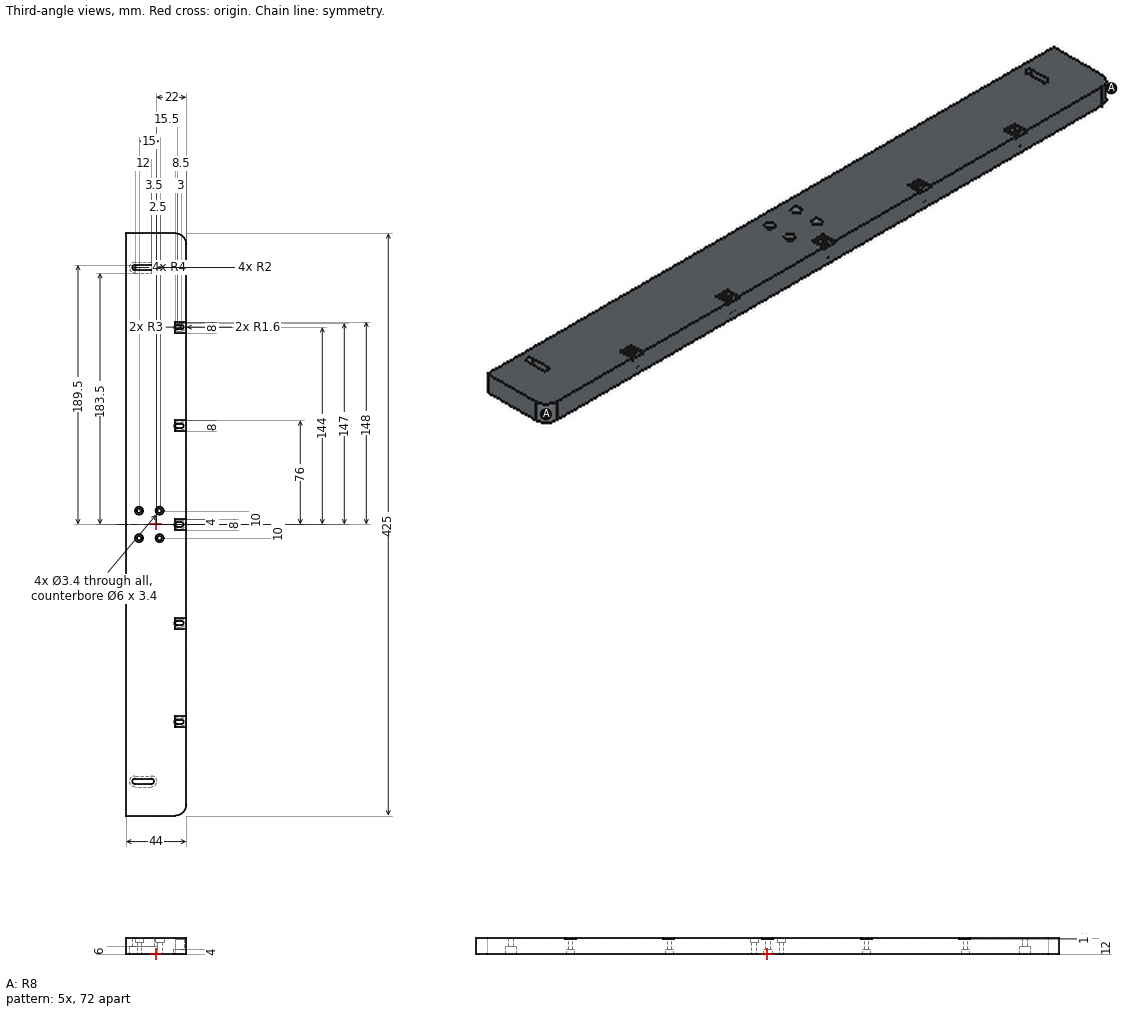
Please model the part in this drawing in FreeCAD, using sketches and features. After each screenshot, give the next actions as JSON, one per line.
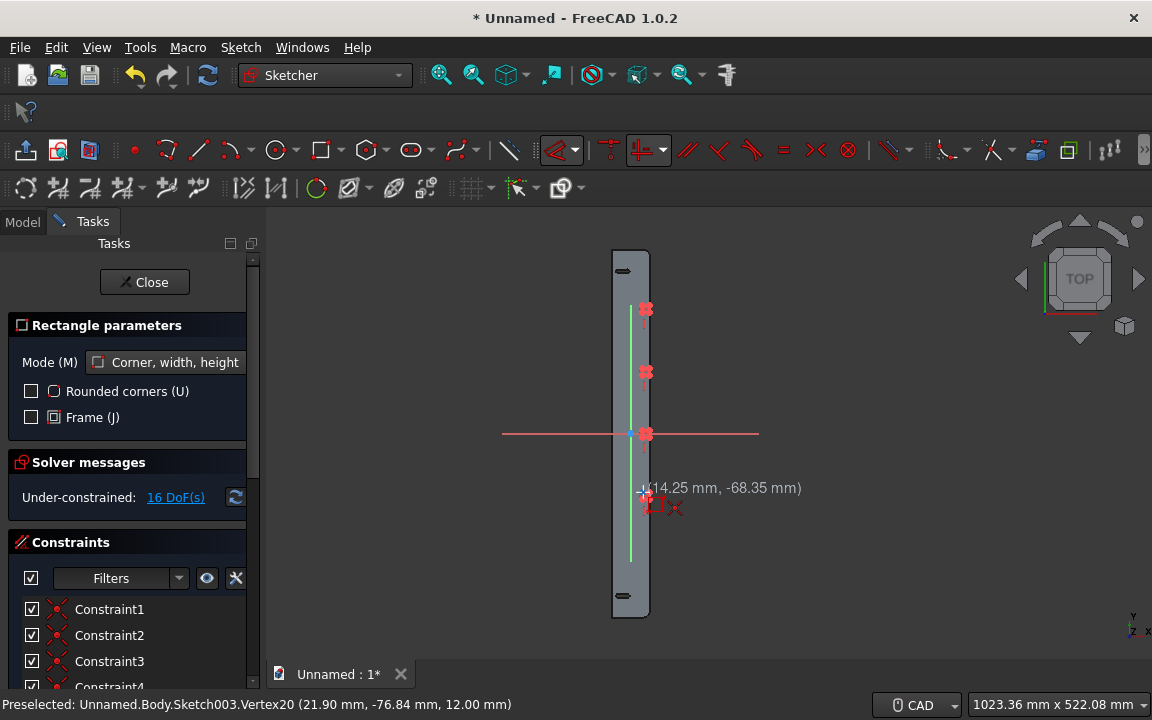
{"action": "scroll", "coordinate": [643, 555], "scroll_direction": "up", "scroll_amount": 5}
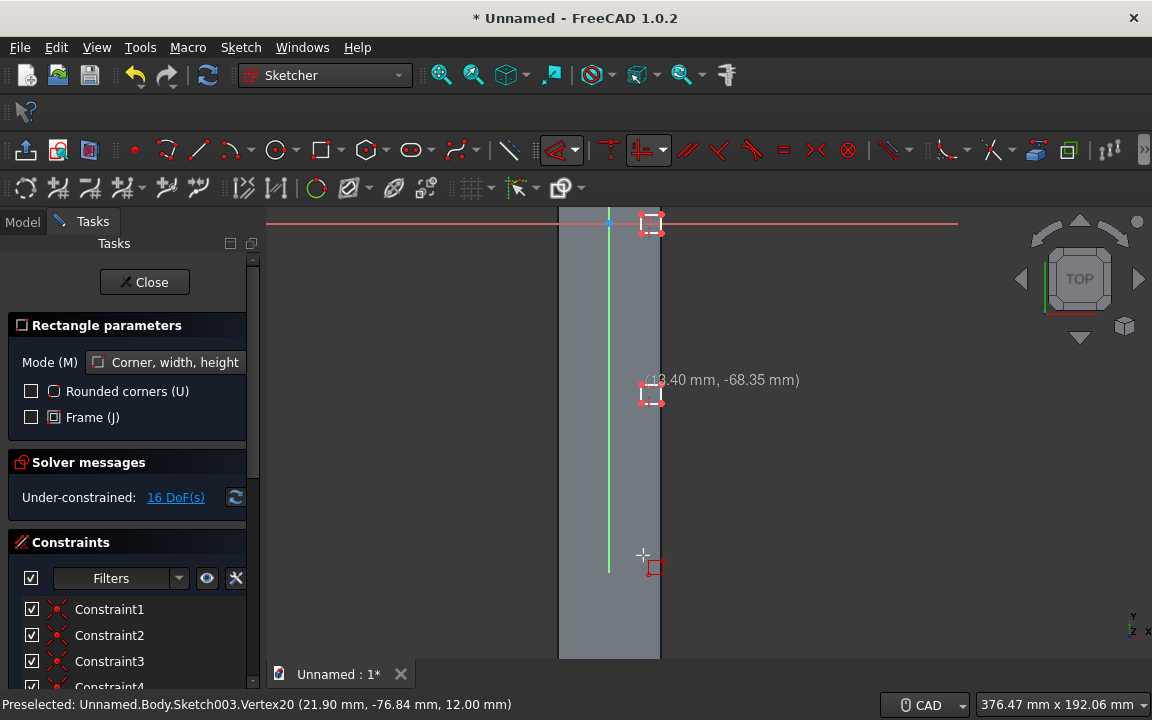
{"action": "left_click", "coordinate": [641, 553]}
{"action": "left_click", "coordinate": [661, 572]}
{"action": "key", "text": "Escape"}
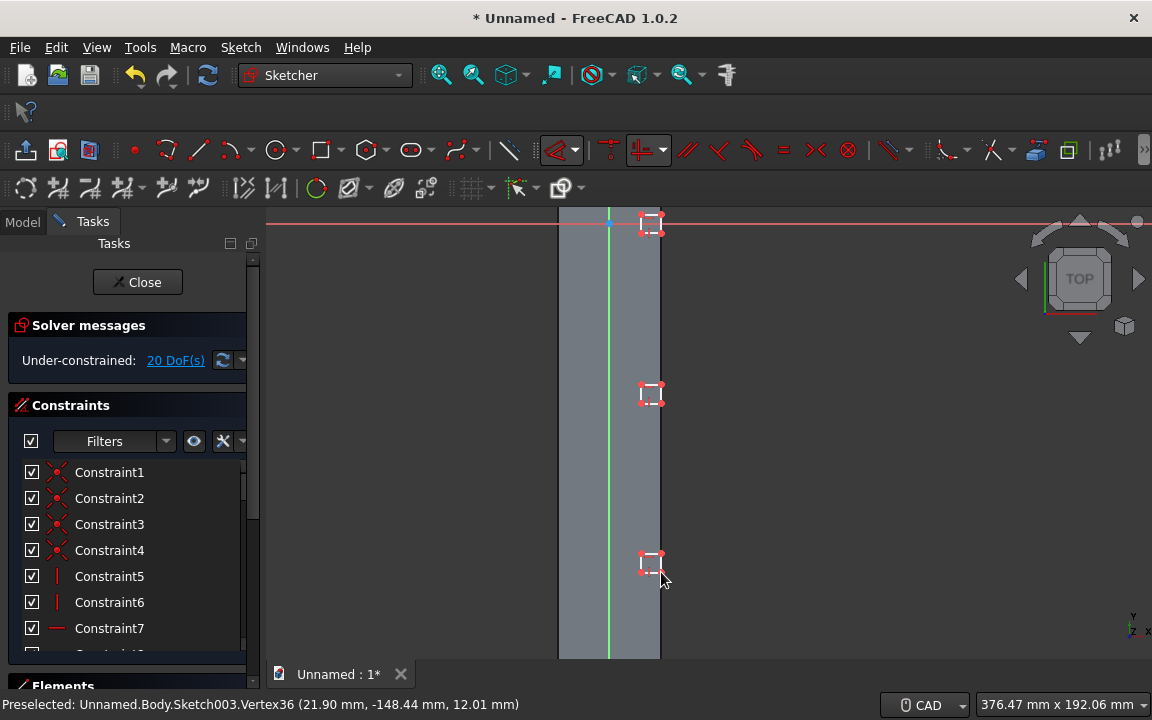
{"action": "scroll", "coordinate": [643, 555], "scroll_direction": "down", "scroll_amount": 5}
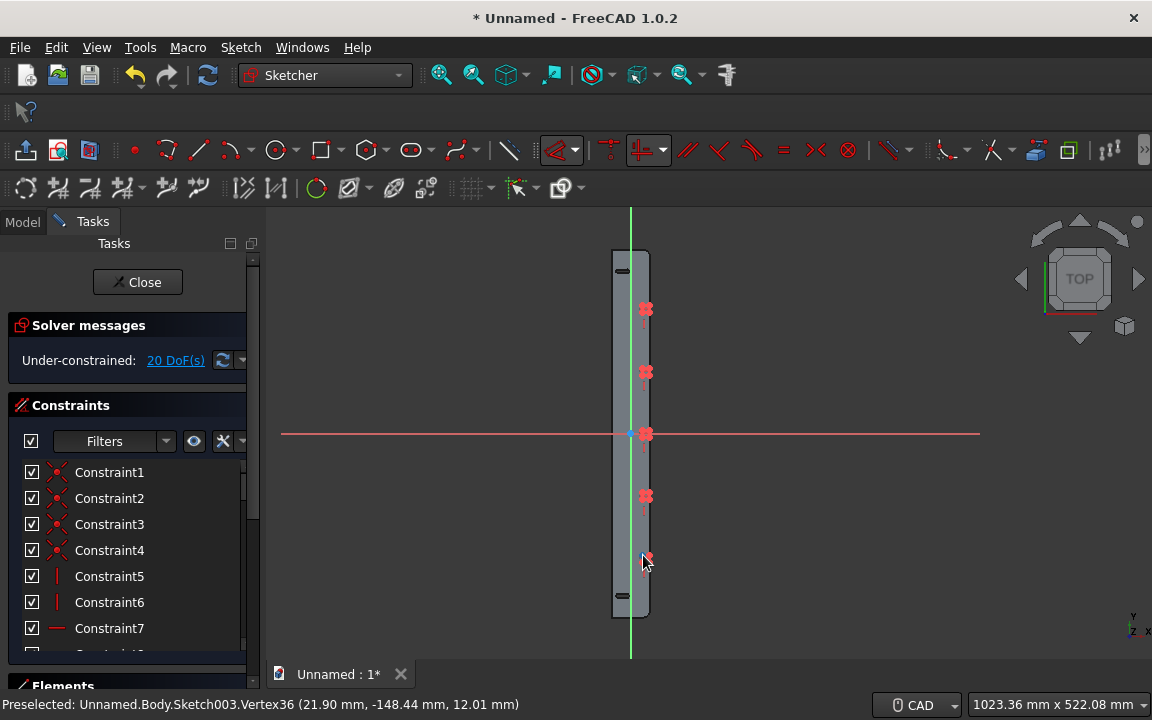
{"action": "scroll", "coordinate": [643, 375], "scroll_direction": "up", "scroll_amount": 3}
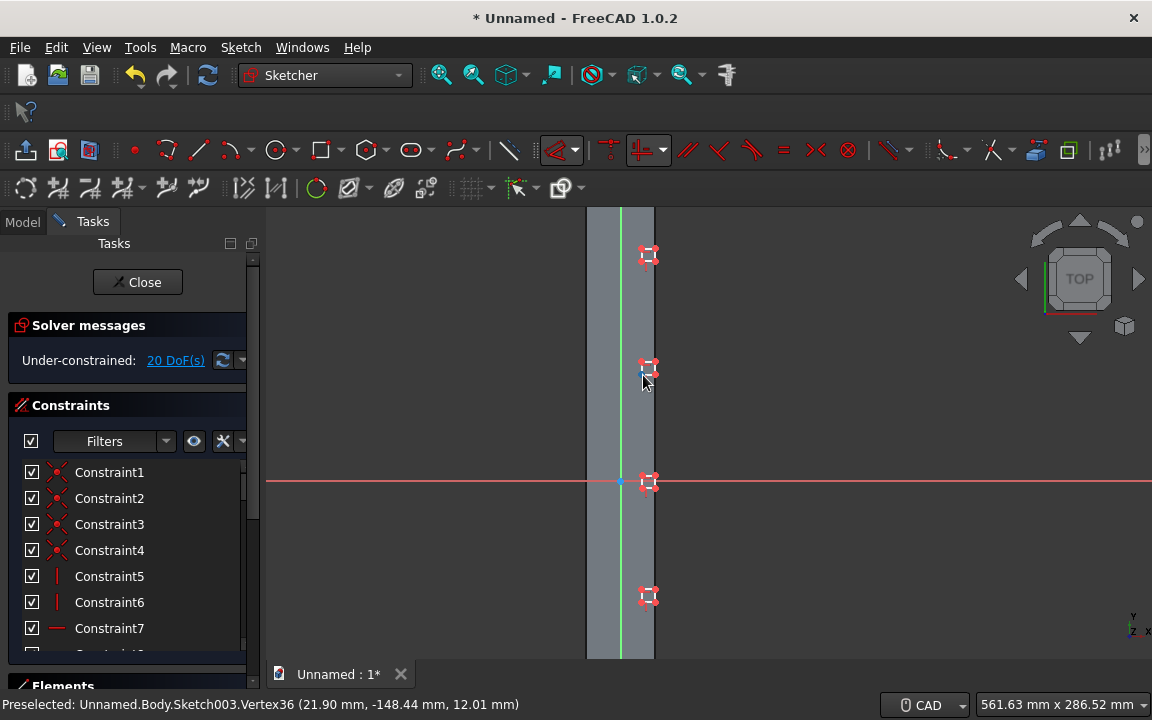
{"action": "left_click", "coordinate": [642, 375]}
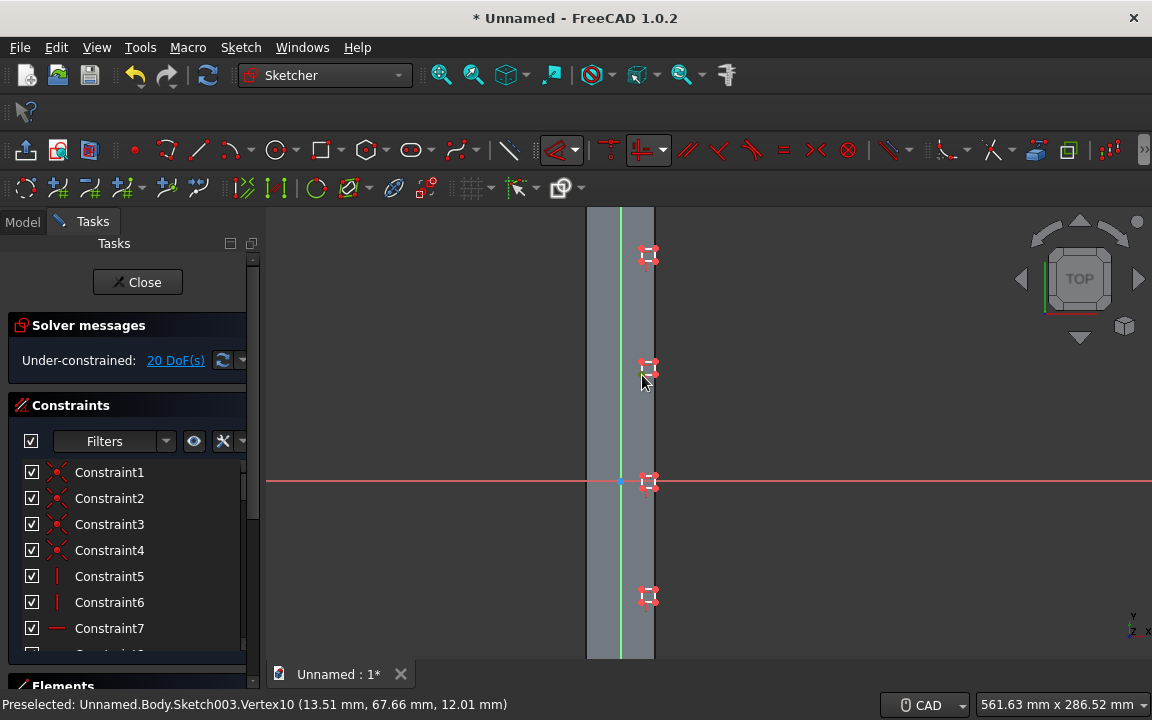
{"action": "left_click", "coordinate": [642, 589]}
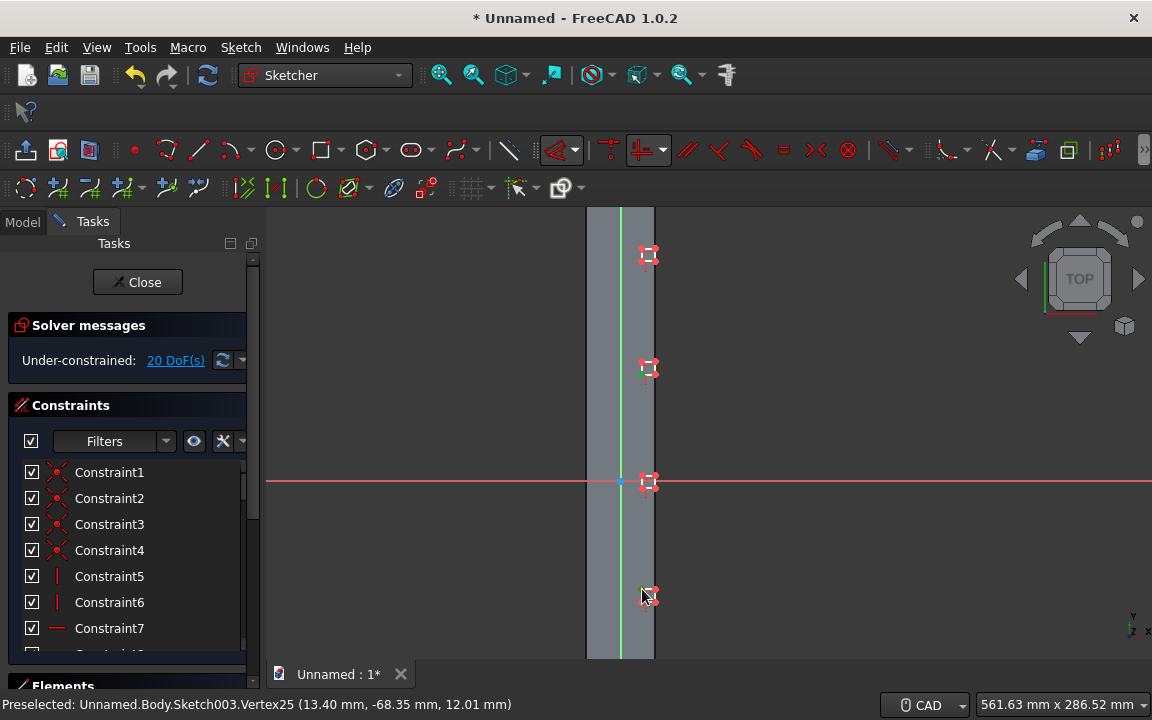
{"action": "left_click", "coordinate": [343, 481]}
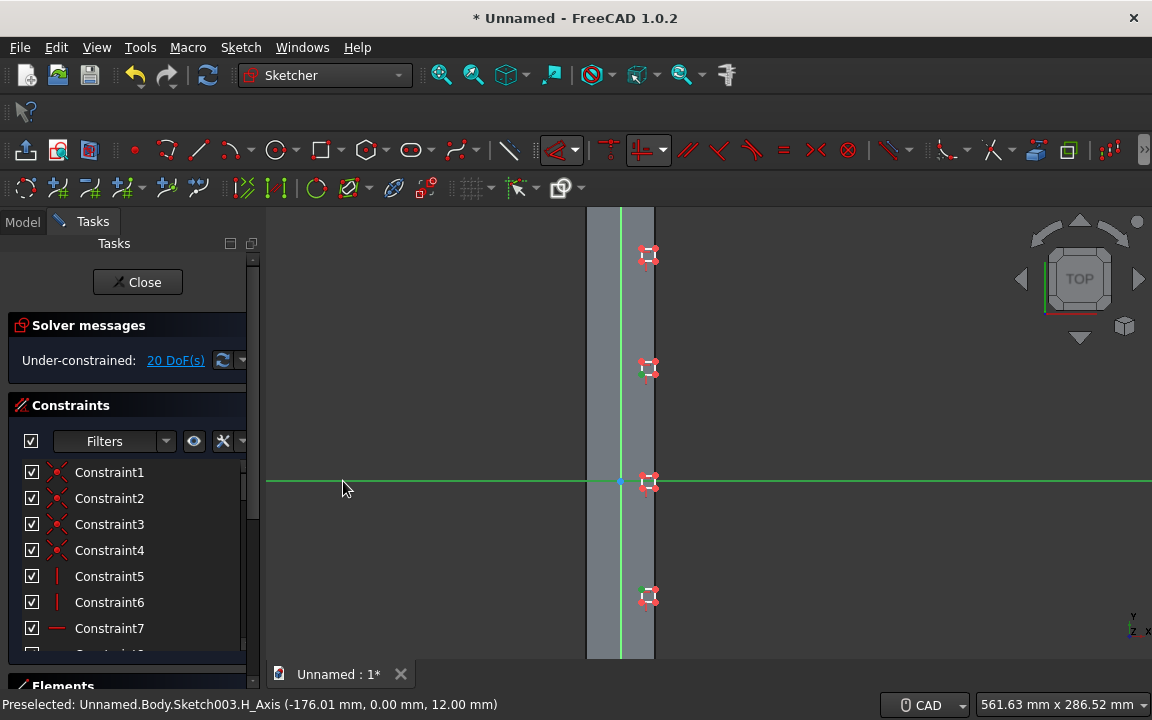
{"action": "left_click", "coordinate": [816, 150]}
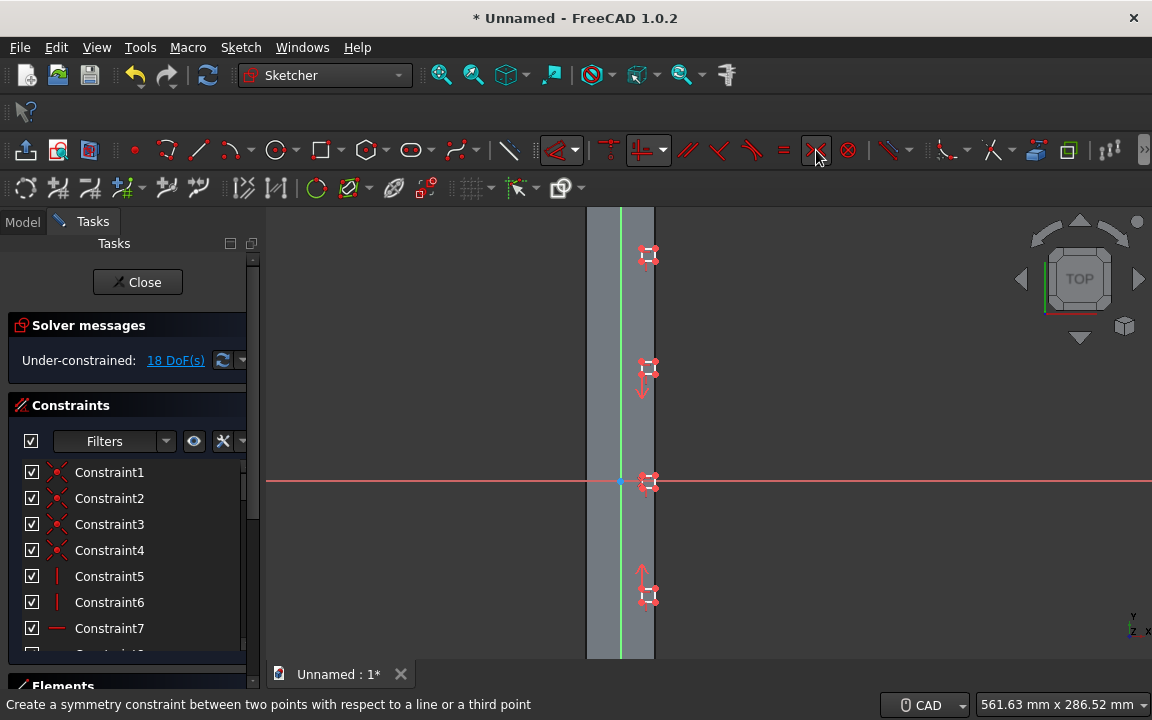
{"action": "left_click", "coordinate": [655, 362]}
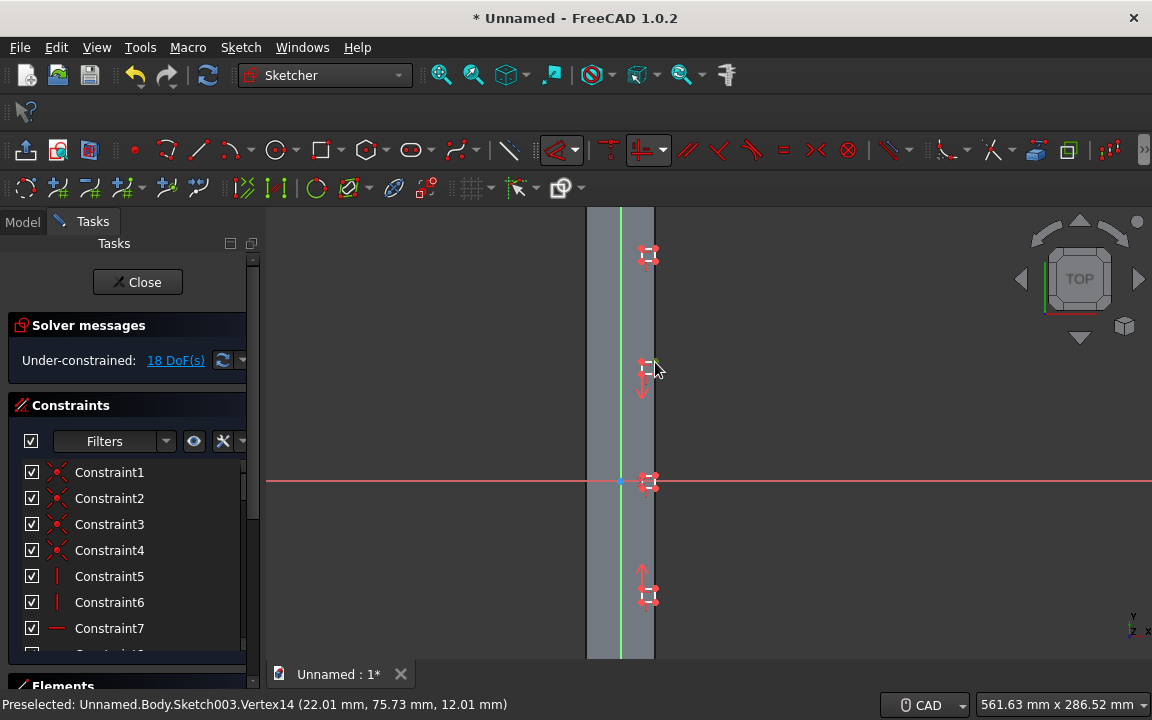
{"action": "left_click", "coordinate": [655, 602]}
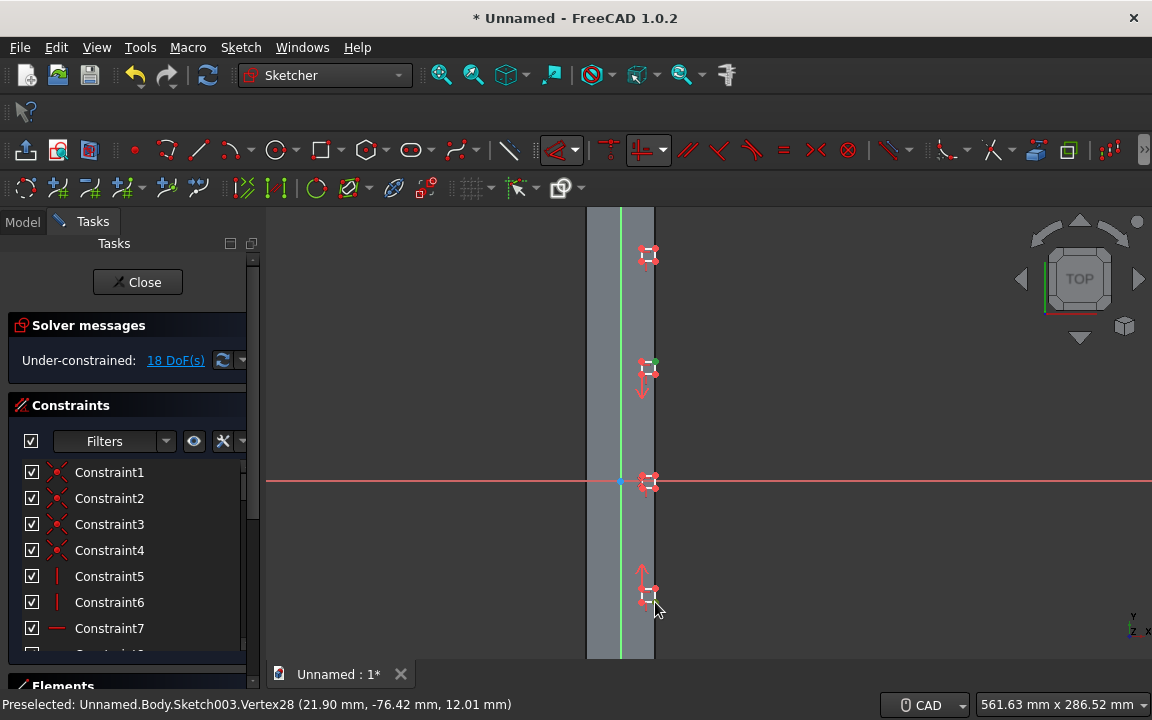
{"action": "left_click", "coordinate": [343, 481]}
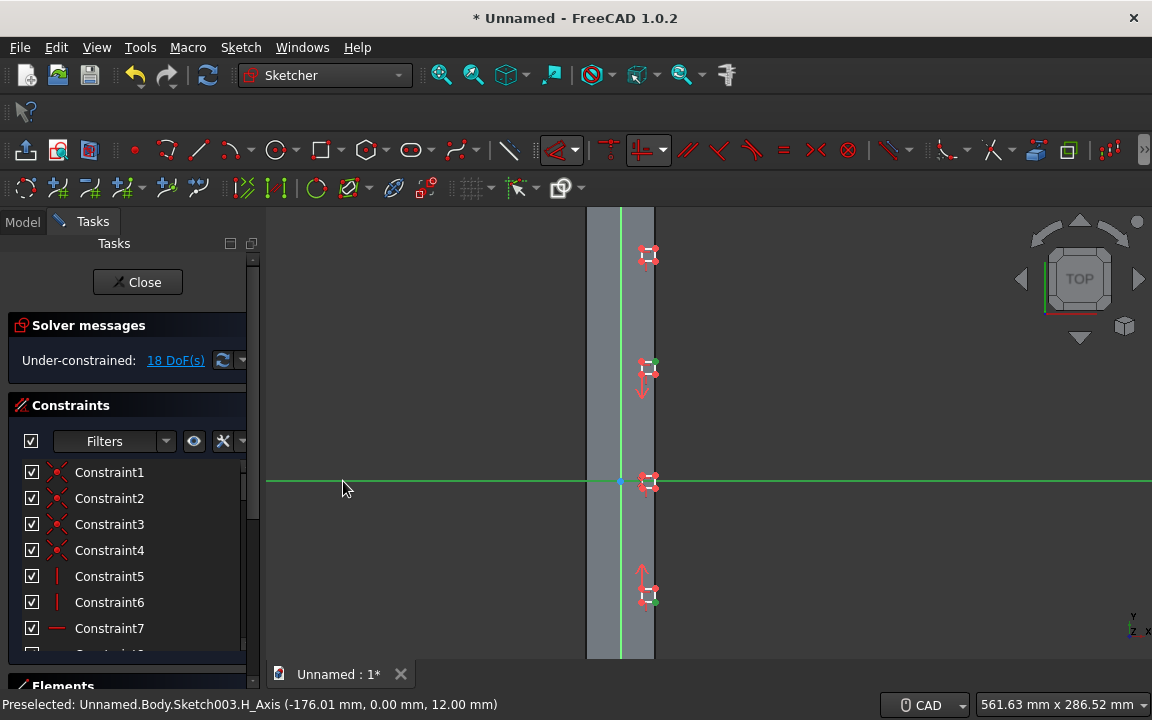
{"action": "left_click", "coordinate": [816, 150]}